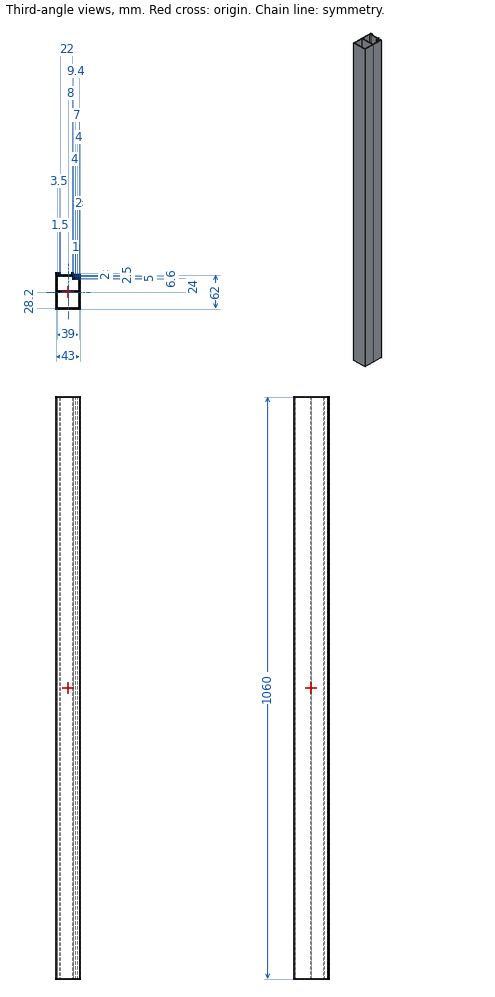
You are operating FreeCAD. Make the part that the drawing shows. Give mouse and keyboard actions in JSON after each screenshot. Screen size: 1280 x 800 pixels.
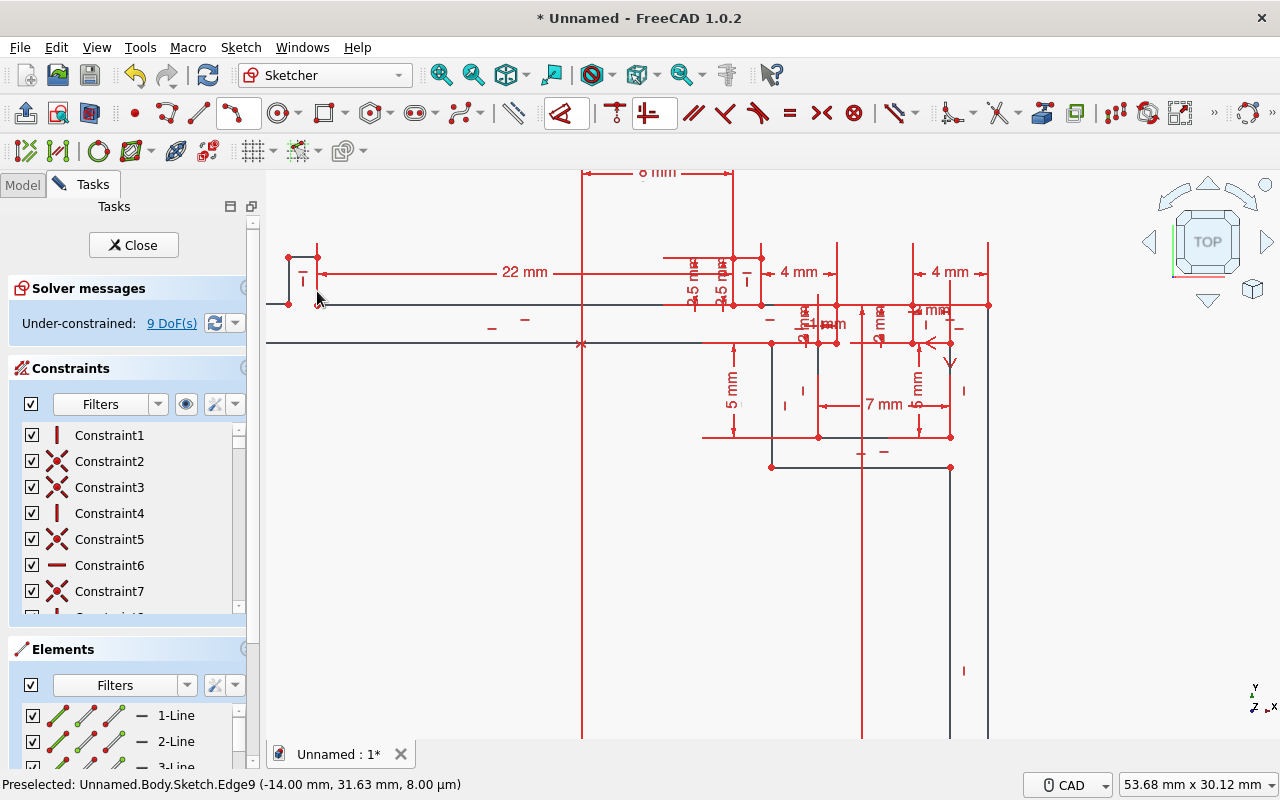
{"action": "left_click", "coordinate": [584, 114]}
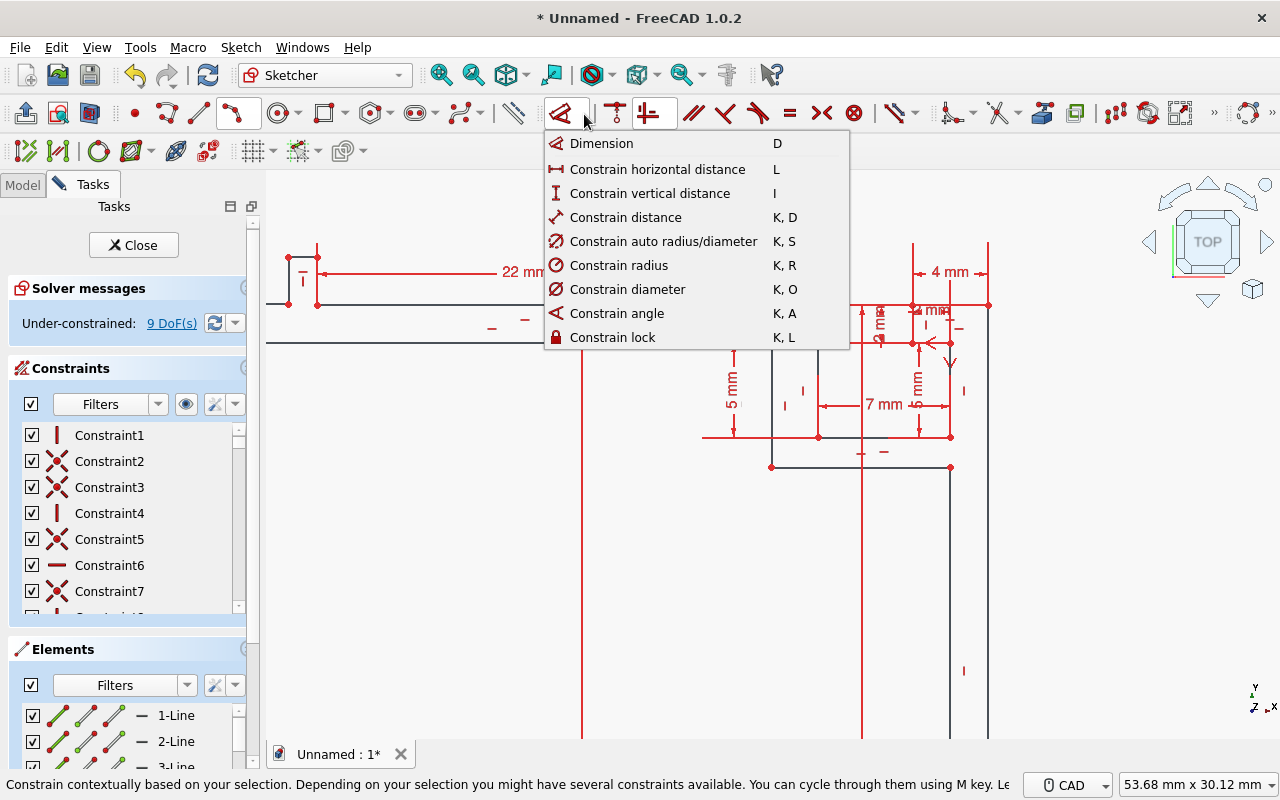
{"action": "left_click", "coordinate": [697, 193]}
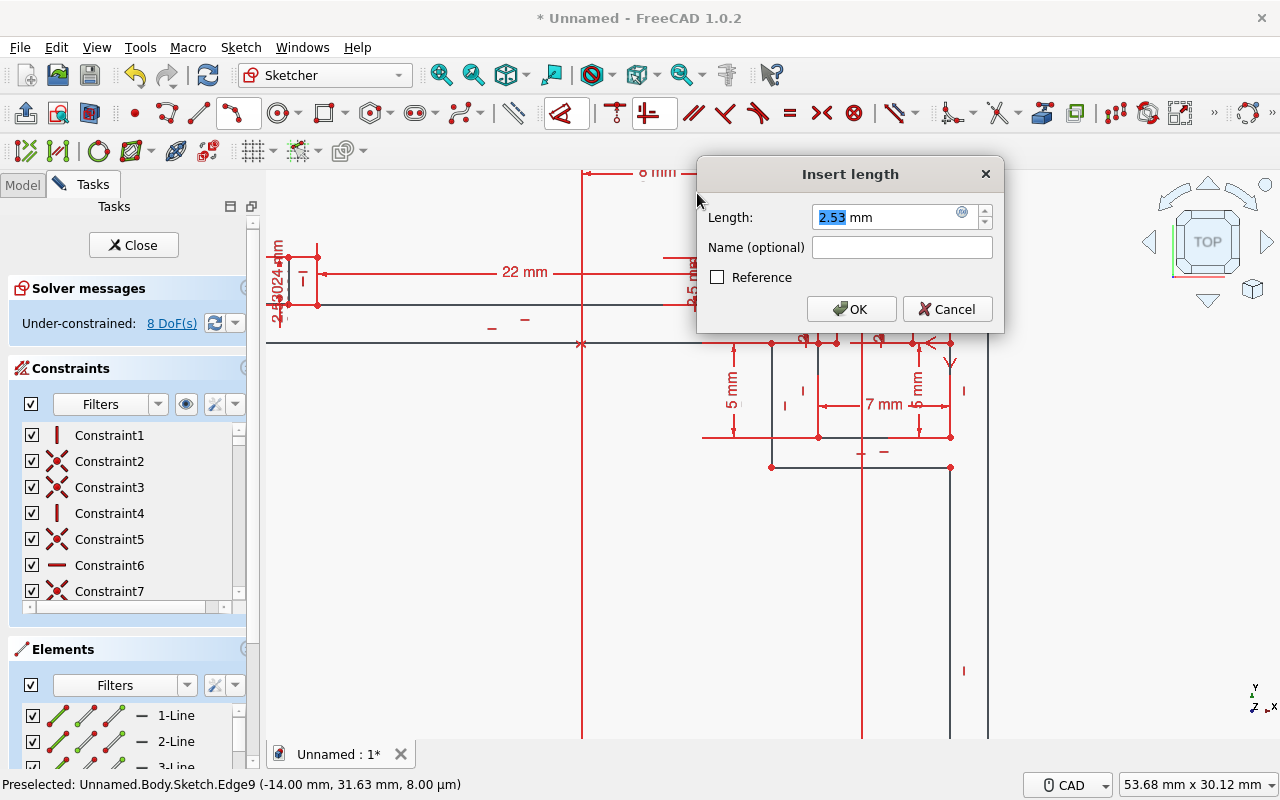
{"action": "type", "text": "2.5"}
{"action": "key", "text": "Return"}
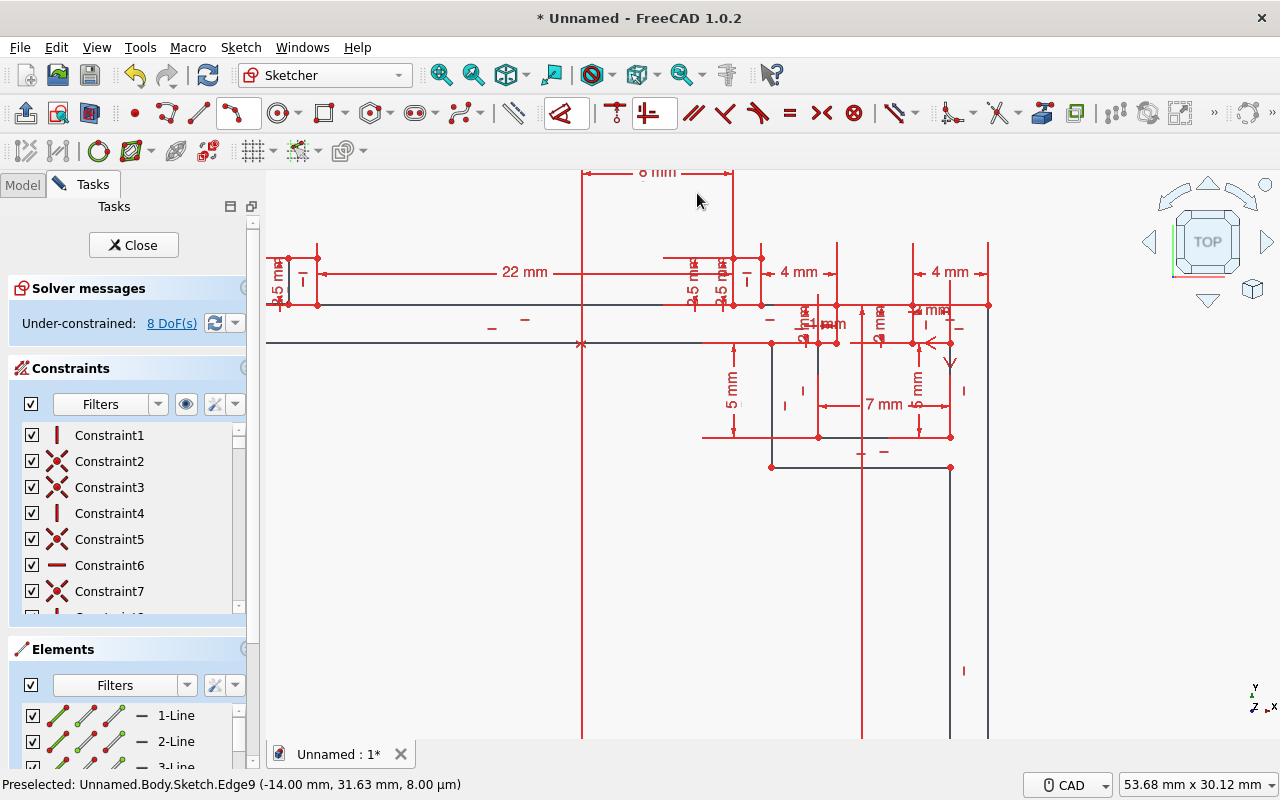
{"action": "scroll", "coordinate": [306, 258], "scroll_direction": "up", "scroll_amount": 2}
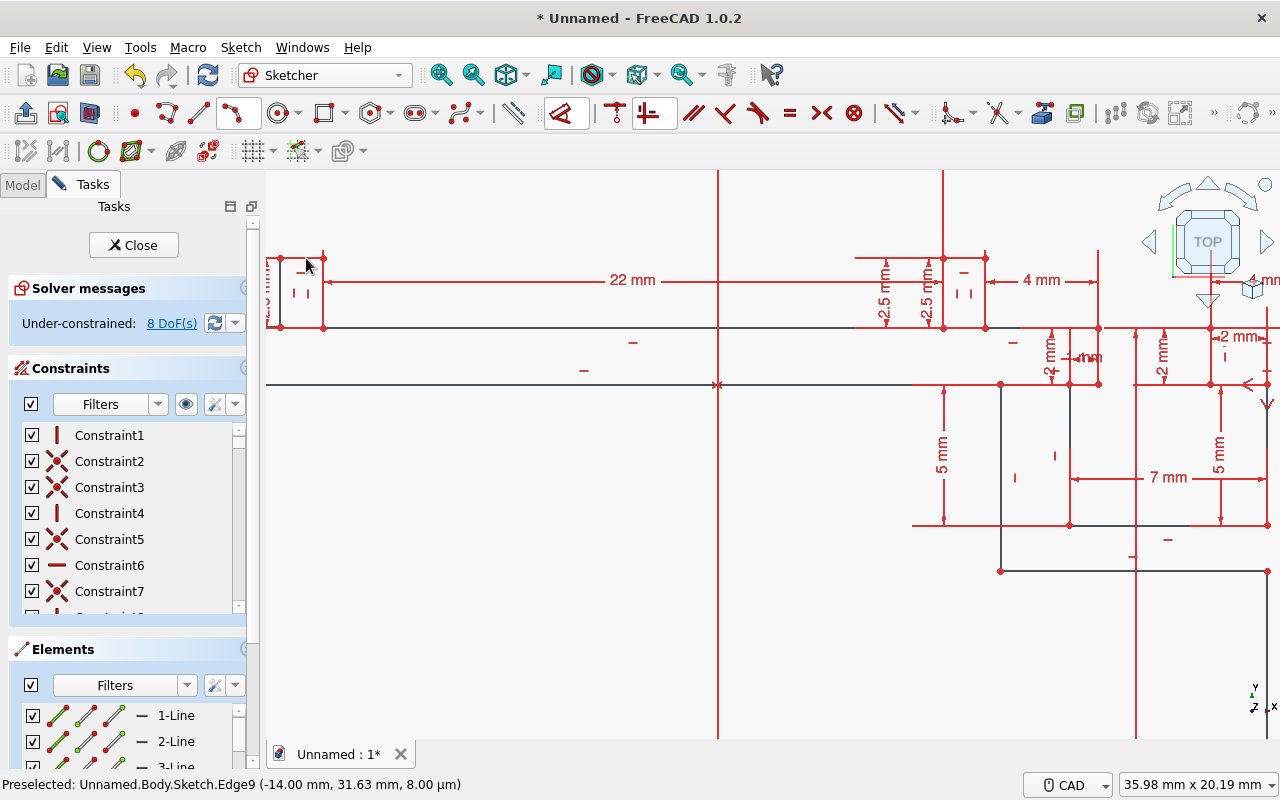
{"action": "left_click", "coordinate": [306, 258]}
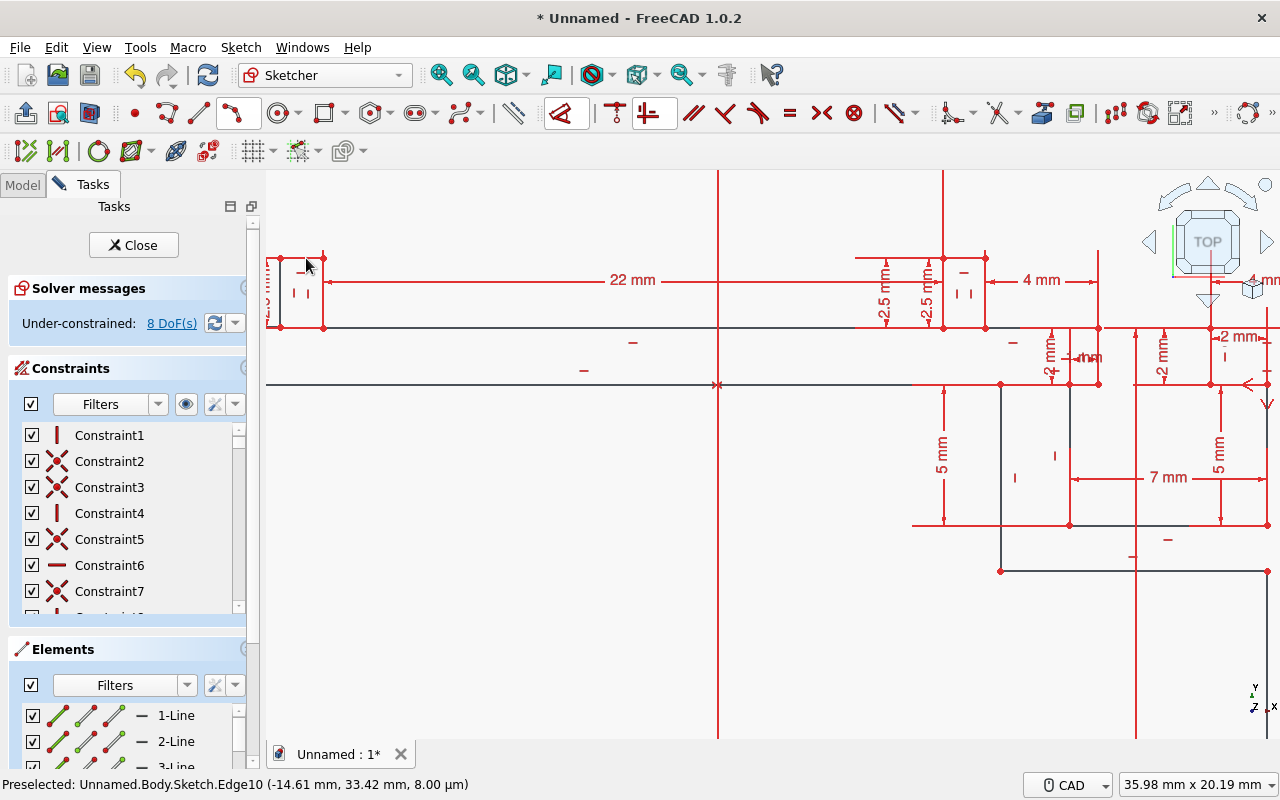
{"action": "left_click", "coordinate": [584, 114]}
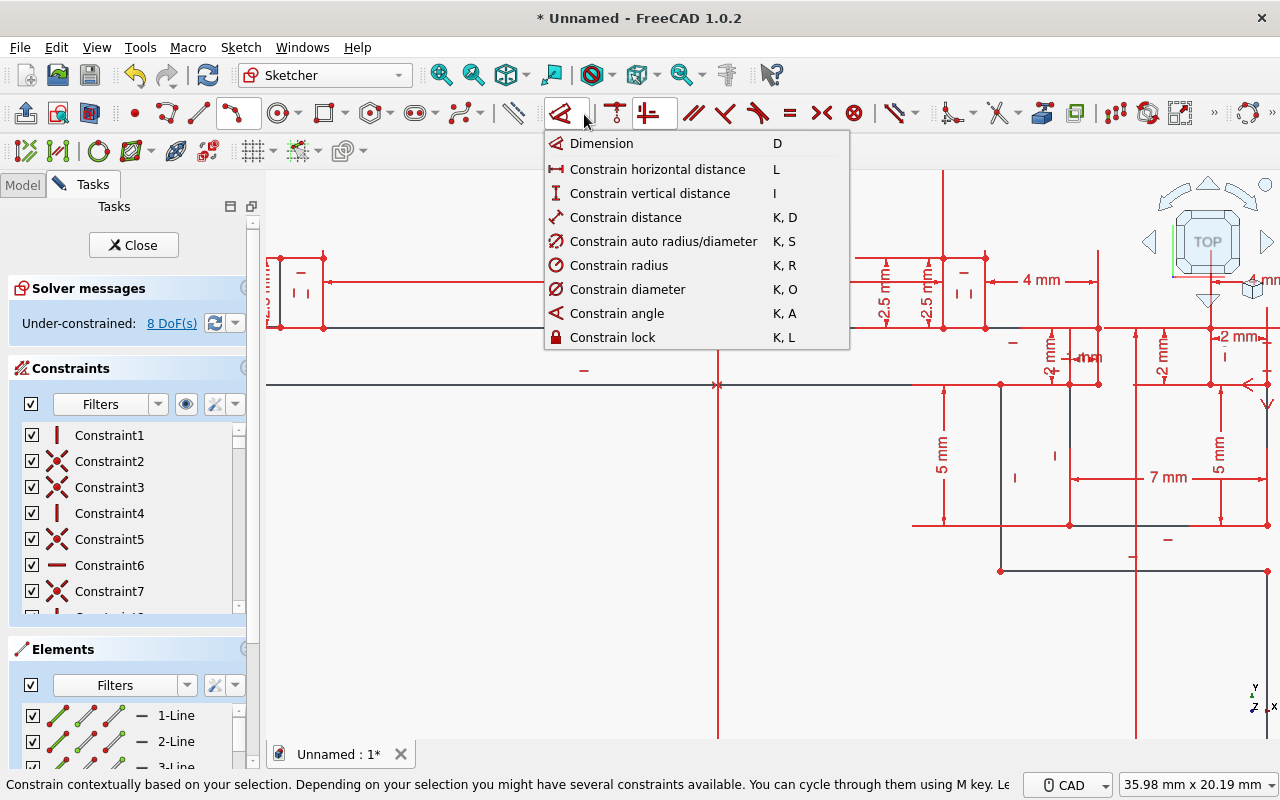
{"action": "left_click", "coordinate": [697, 169]}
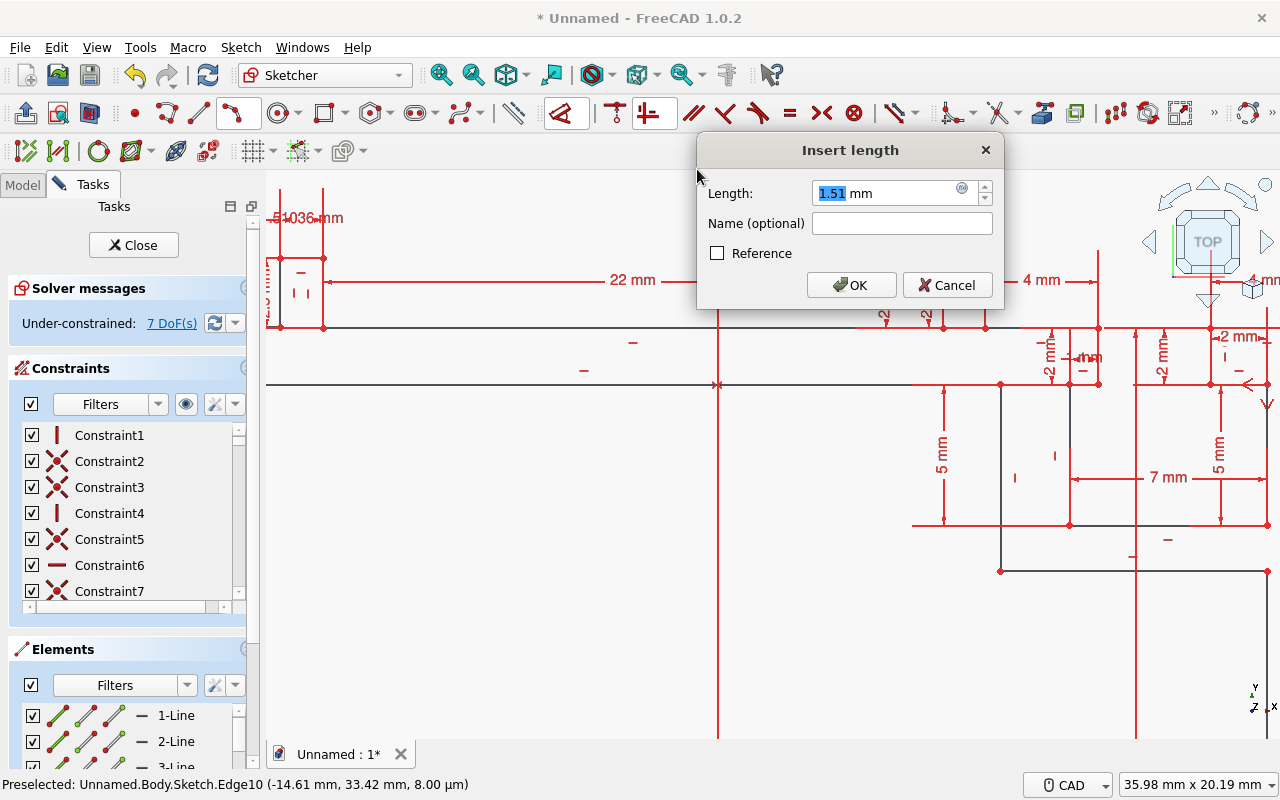
{"action": "type", "text": "1.5"}
{"action": "key", "text": "Return"}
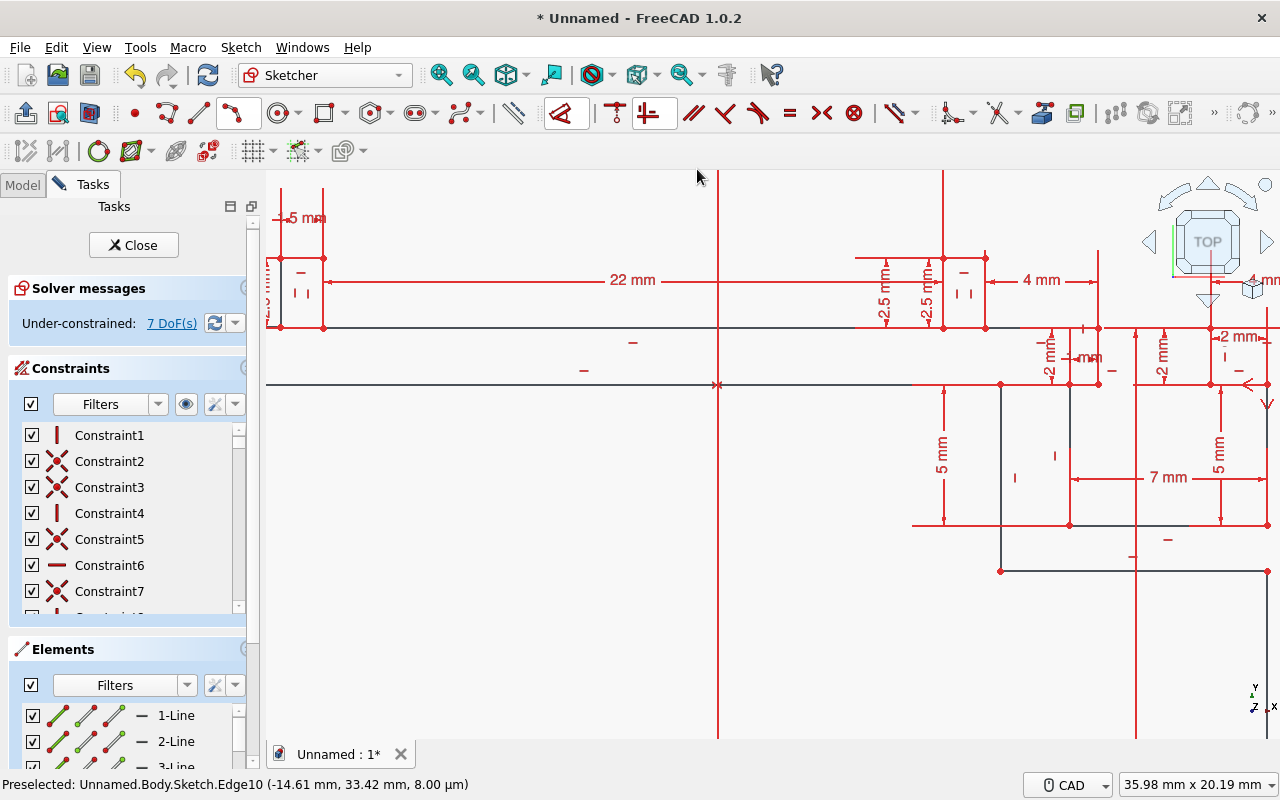
{"action": "scroll", "coordinate": [701, 275], "scroll_direction": "down", "scroll_amount": 8}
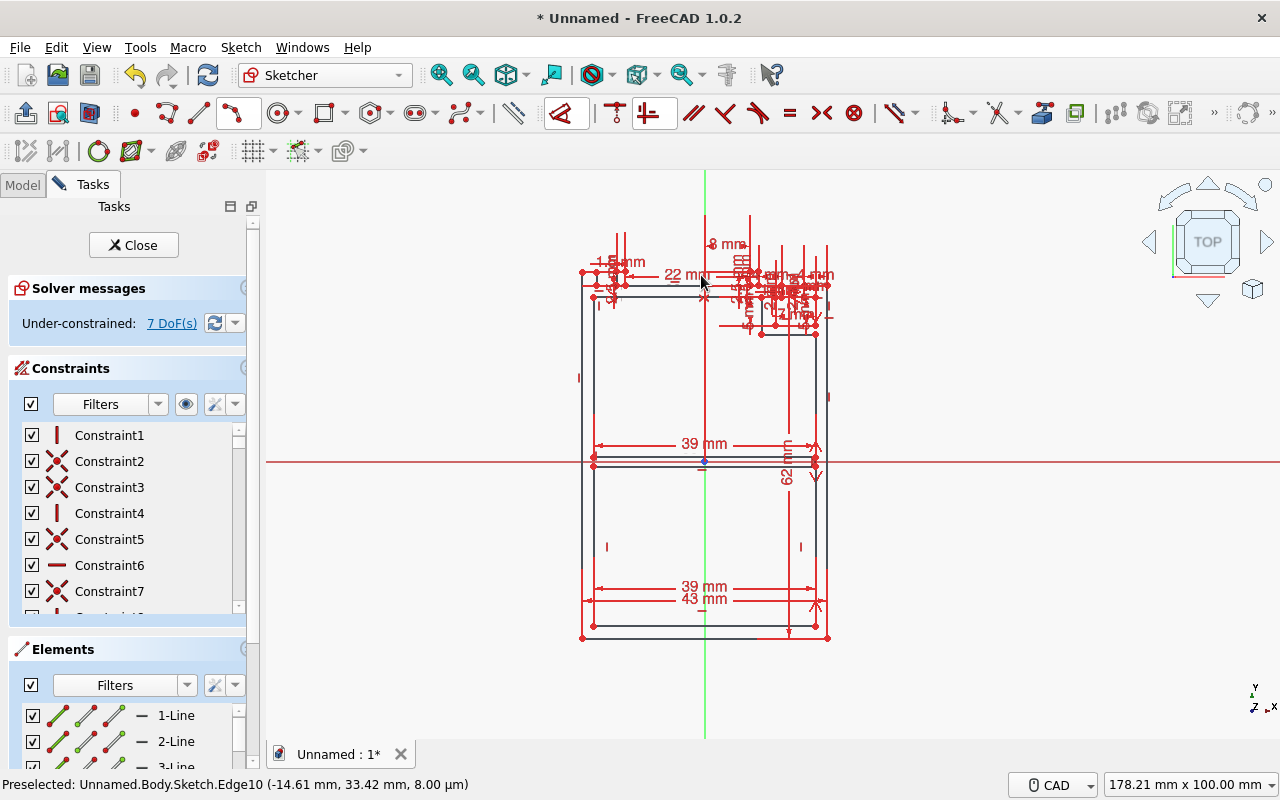
{"action": "scroll", "coordinate": [617, 276], "scroll_direction": "up", "scroll_amount": 6}